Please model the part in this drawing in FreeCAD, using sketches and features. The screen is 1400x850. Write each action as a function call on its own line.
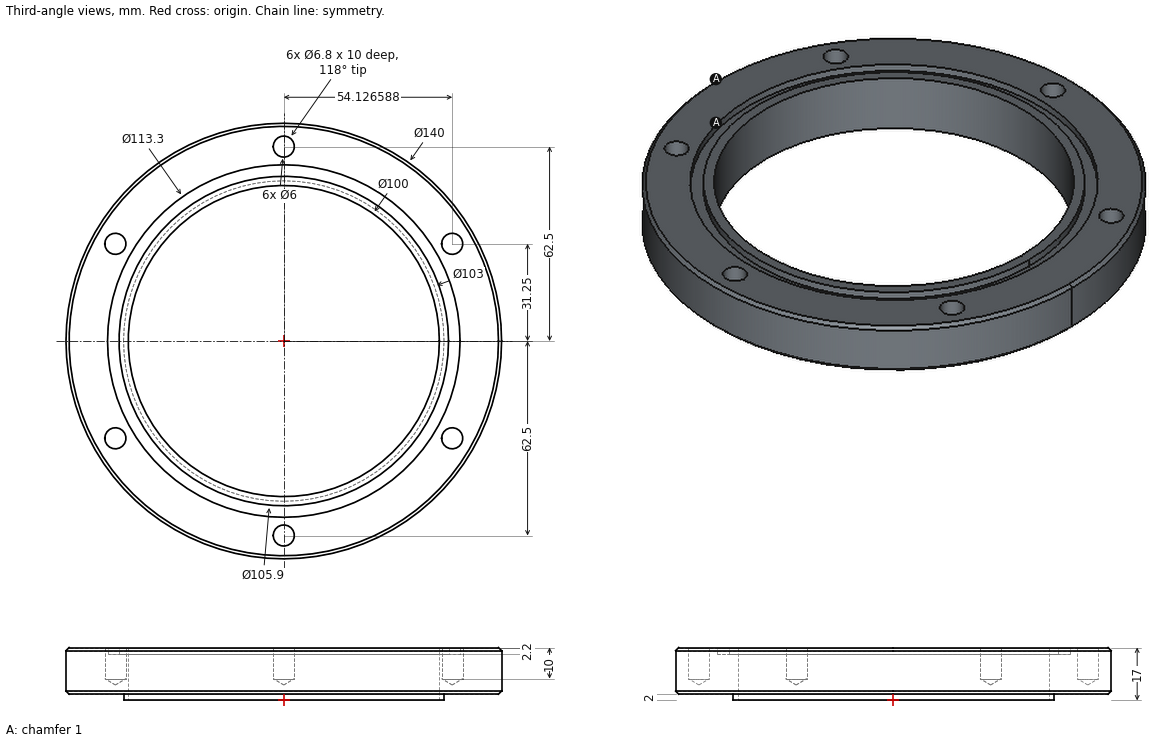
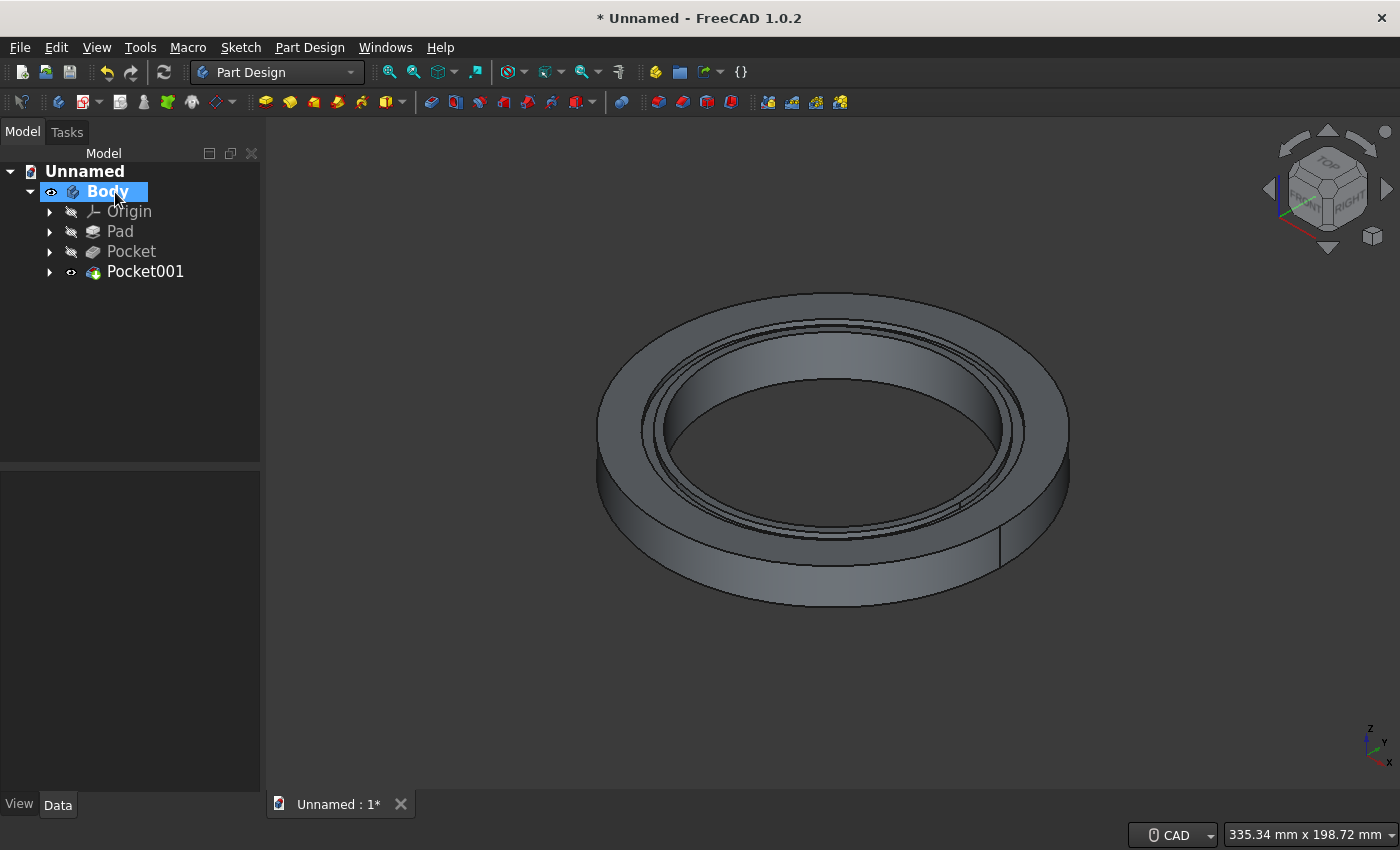
click(1024, 373)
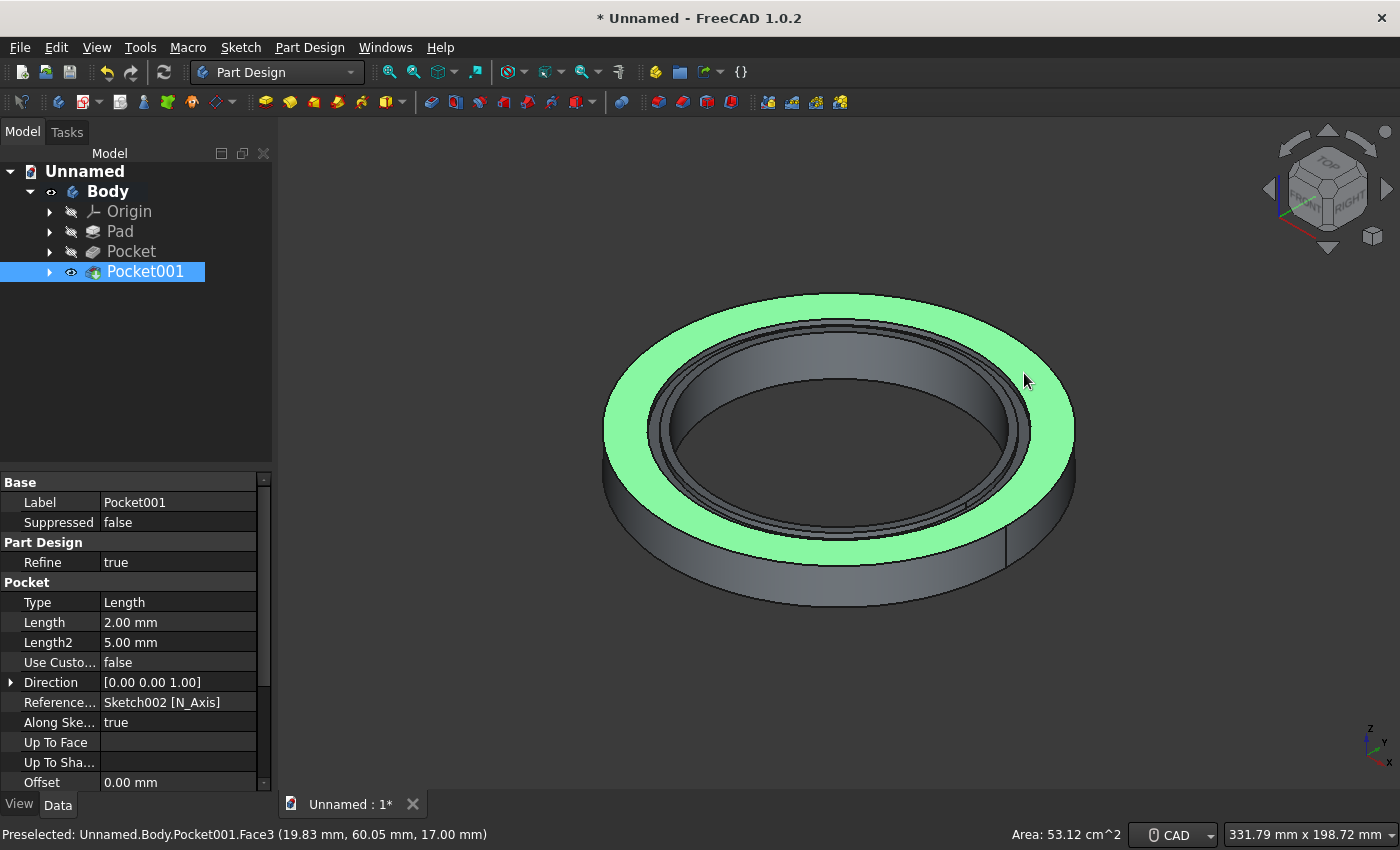
click(84, 102)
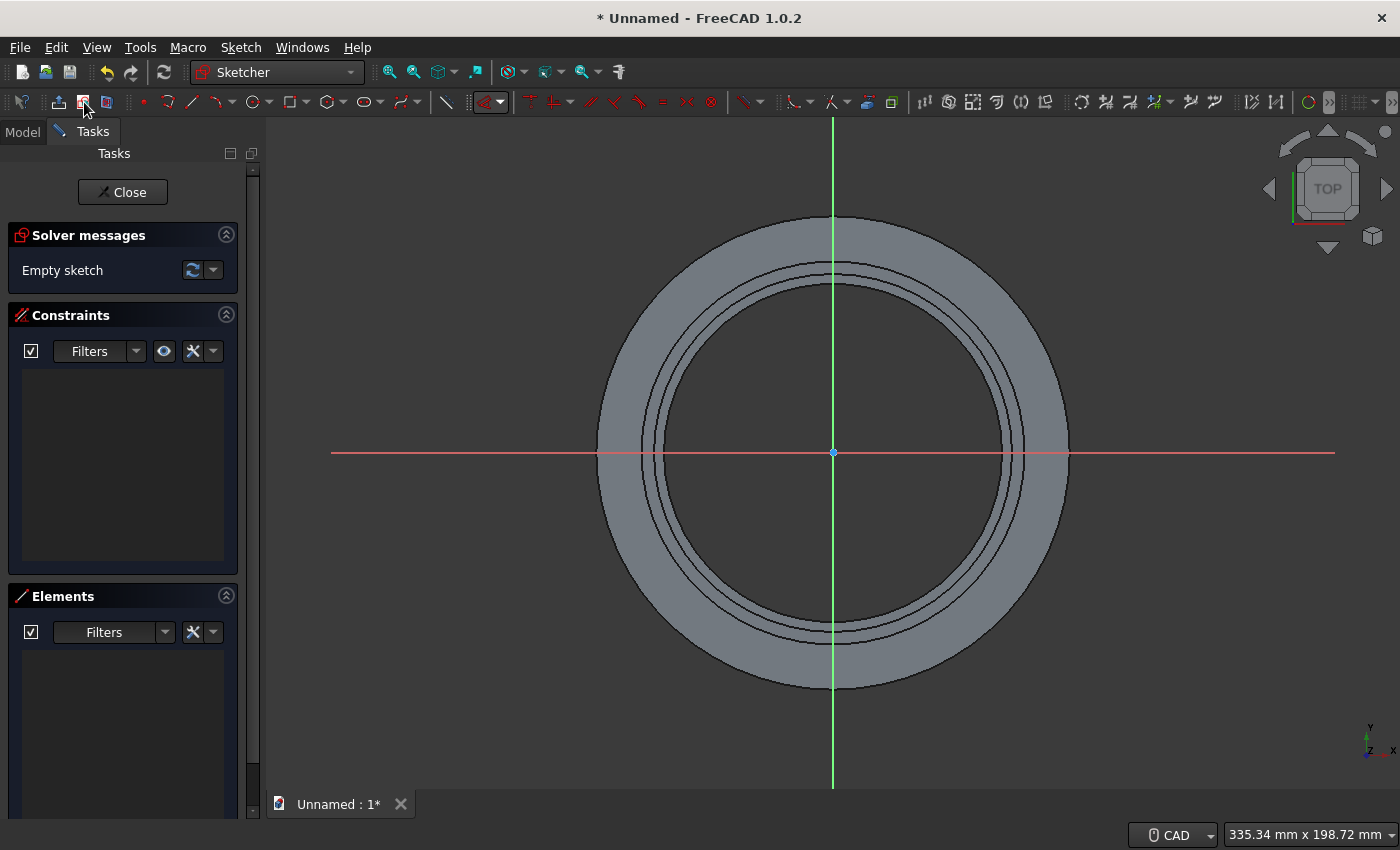
click(254, 102)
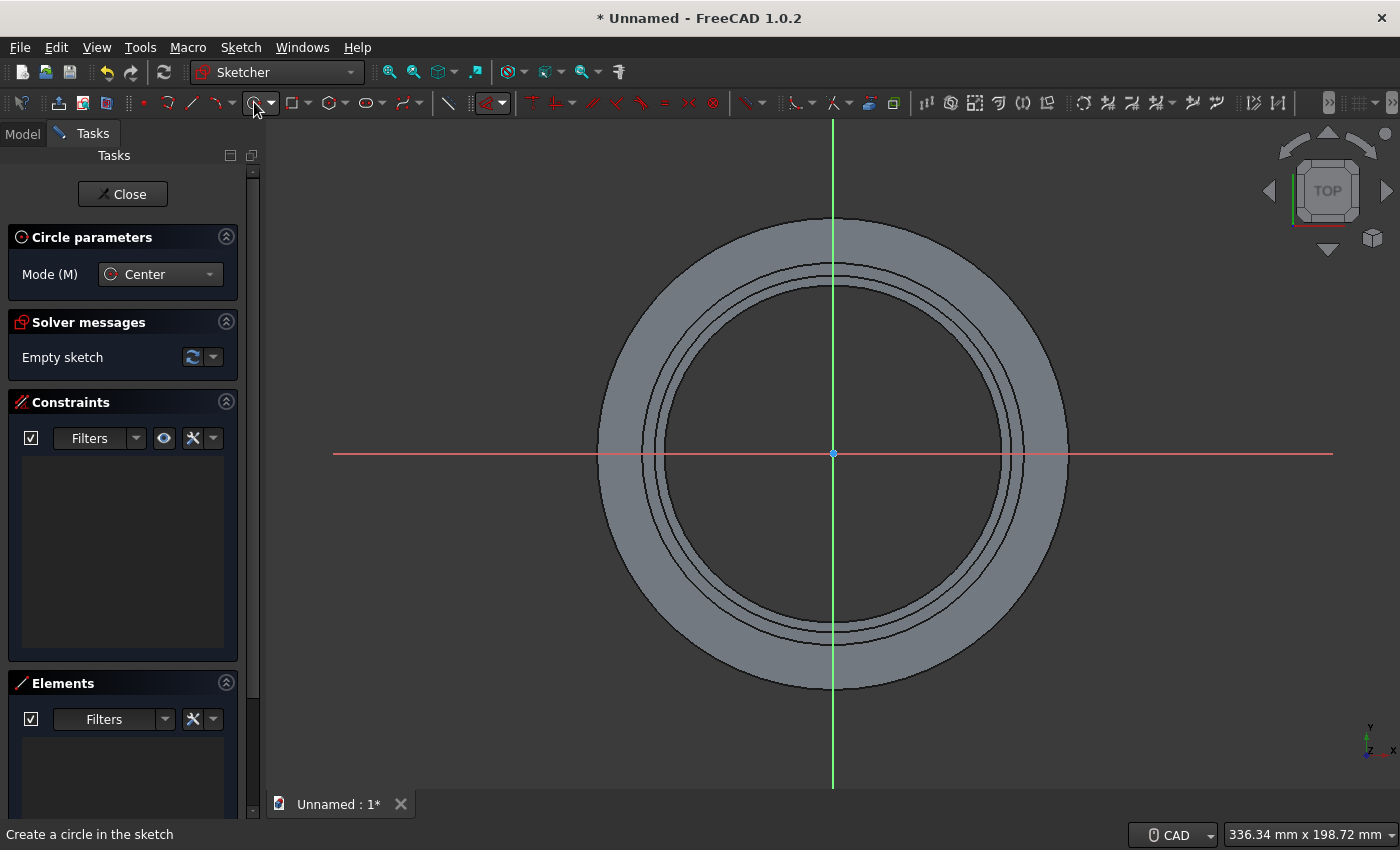
scroll(833, 243, up, 5)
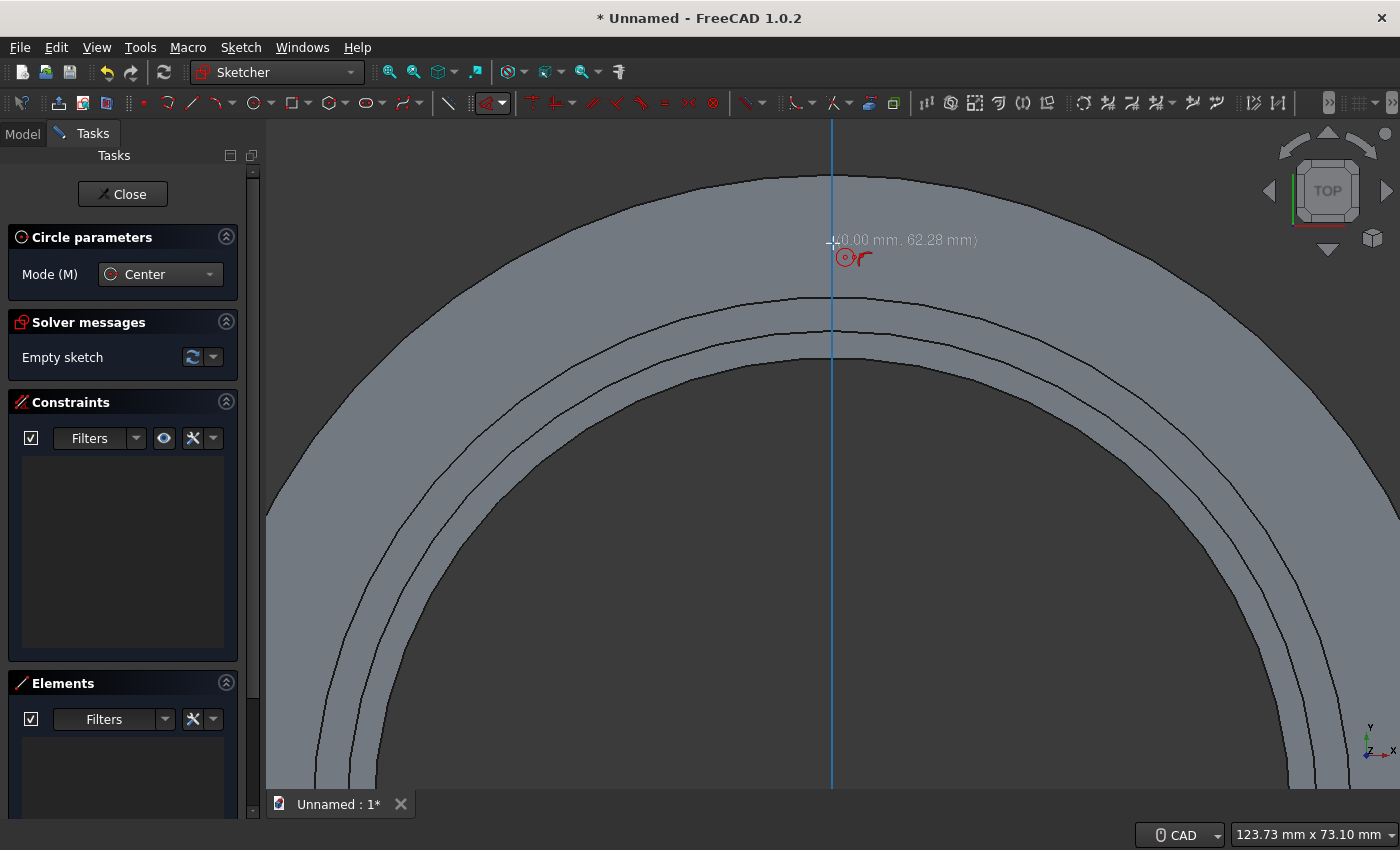
click(832, 243)
move(852, 224)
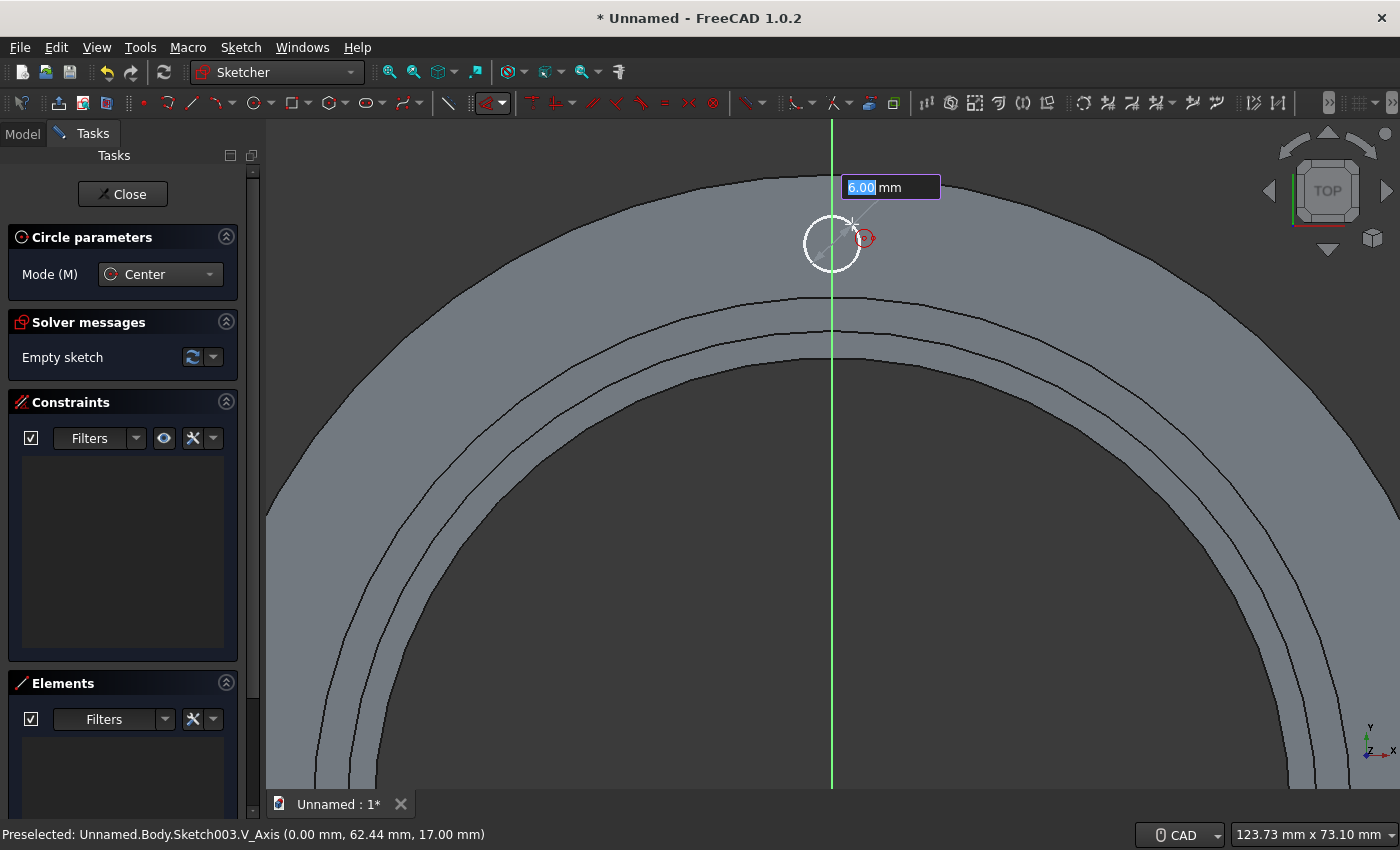
text(6)
key(Return)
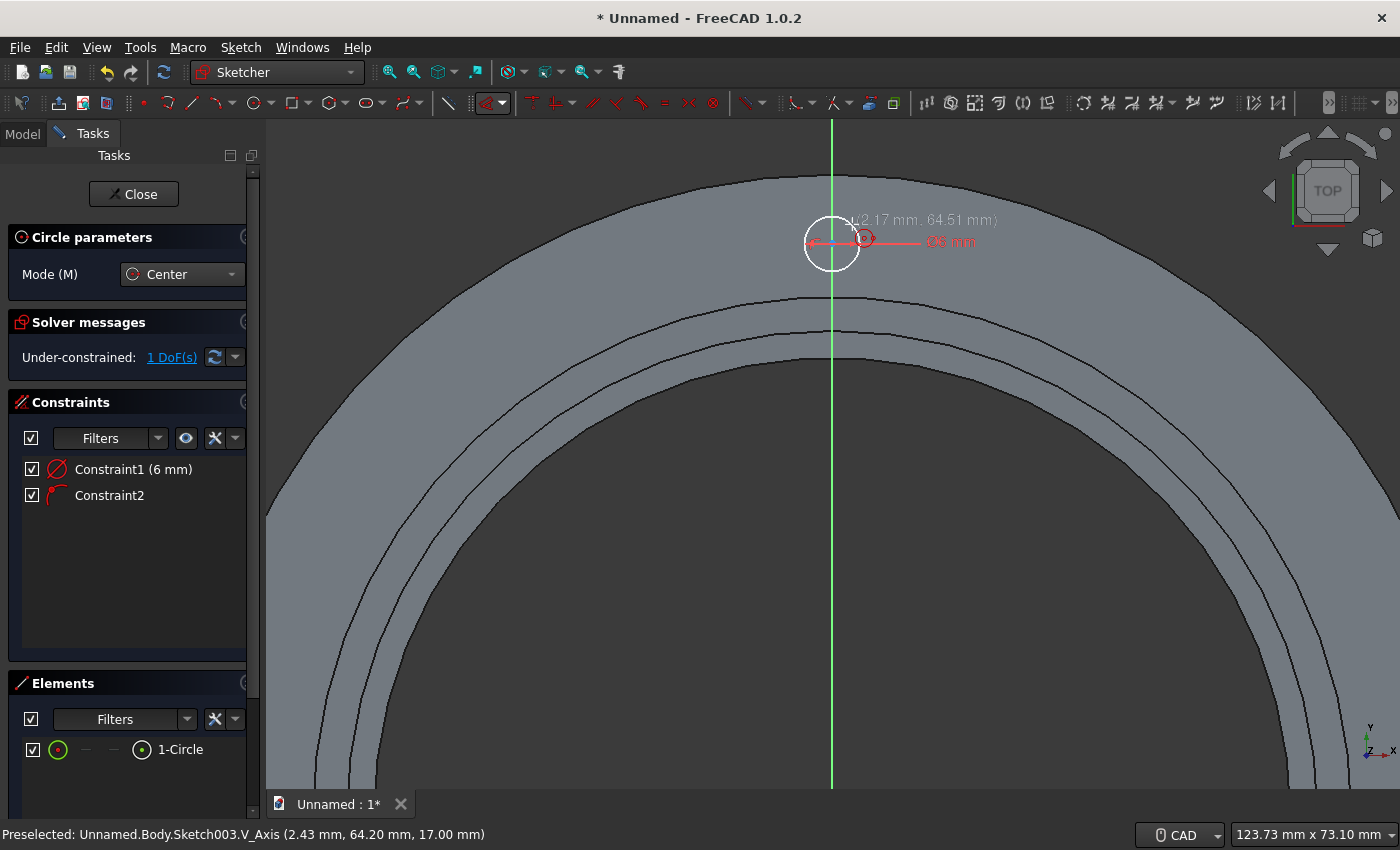
scroll(725, 243, down, 5)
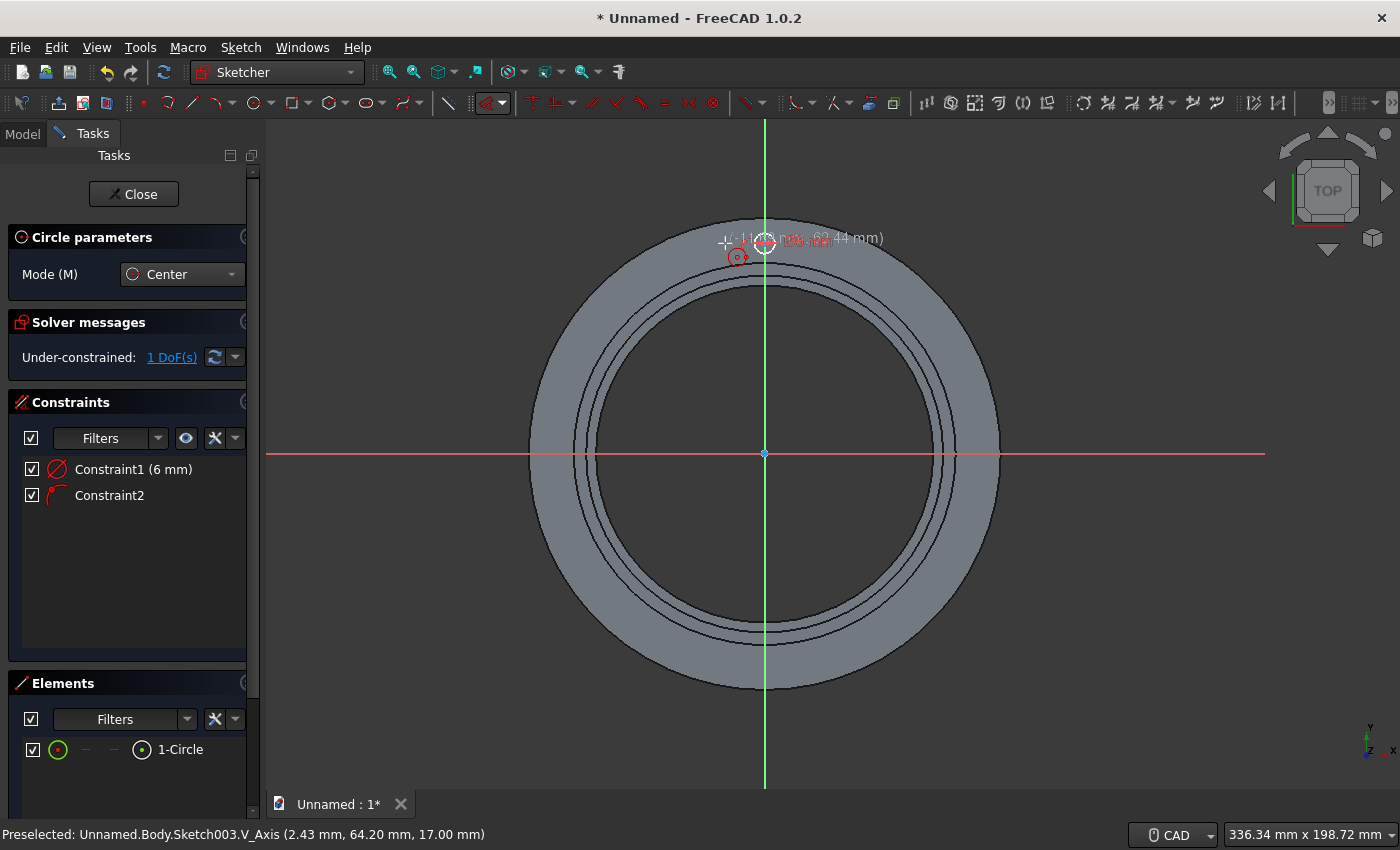
scroll(947, 349, up, 5)